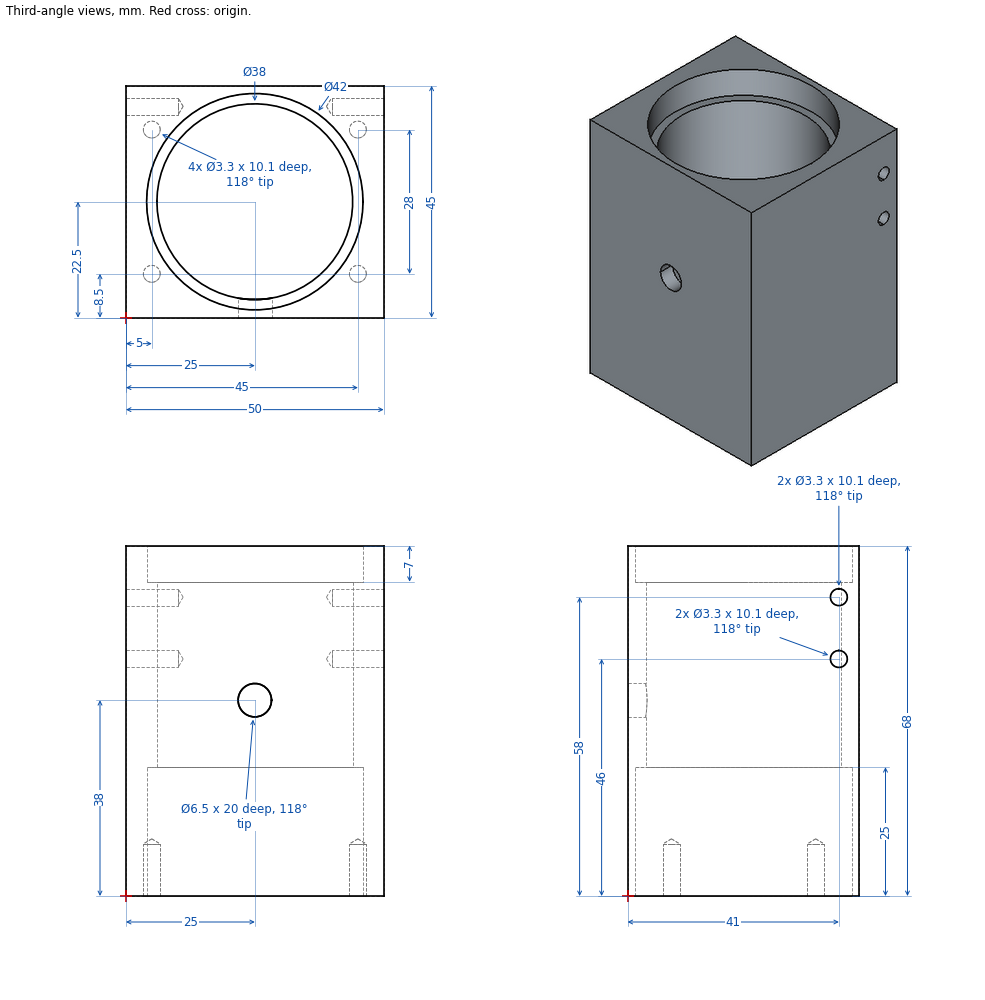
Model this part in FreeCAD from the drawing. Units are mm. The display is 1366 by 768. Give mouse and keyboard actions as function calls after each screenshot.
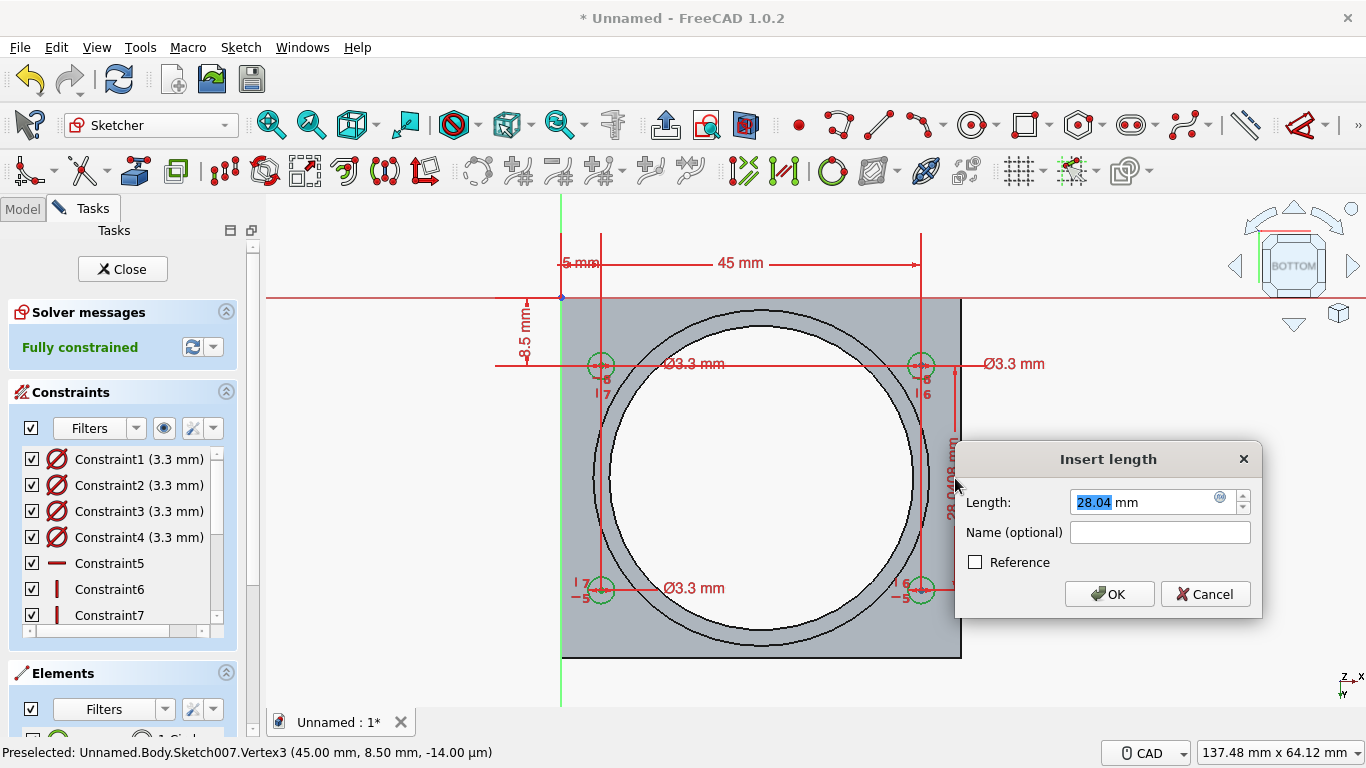
text(28)
key(Return)
key(Escape)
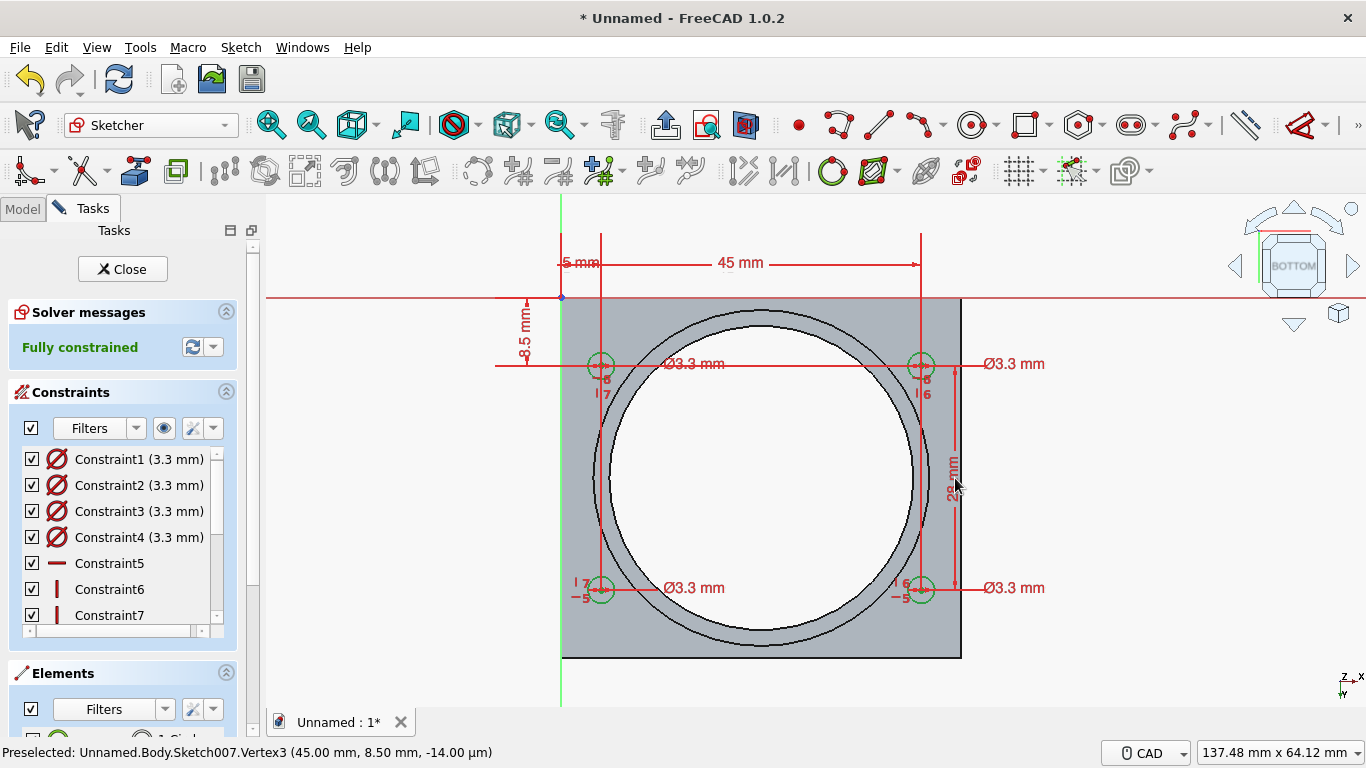
click(123, 269)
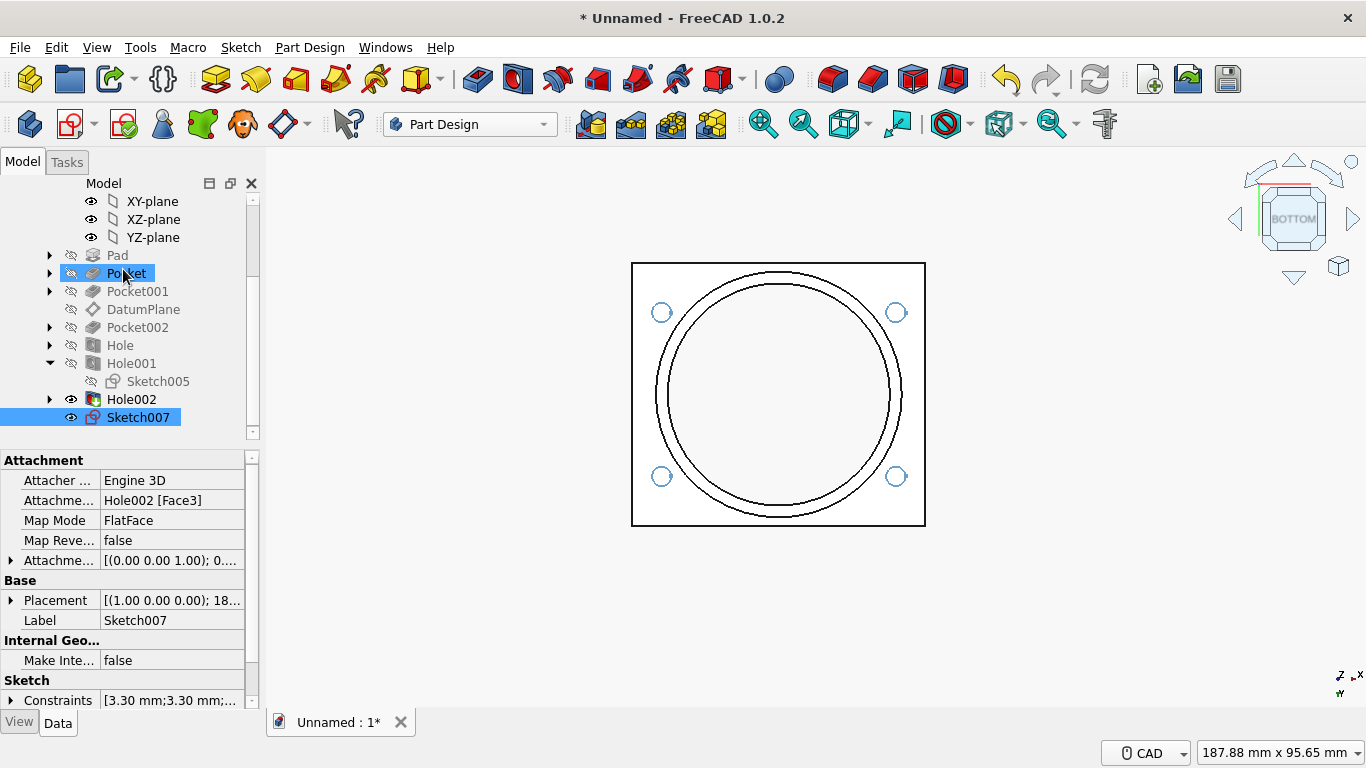
click(518, 80)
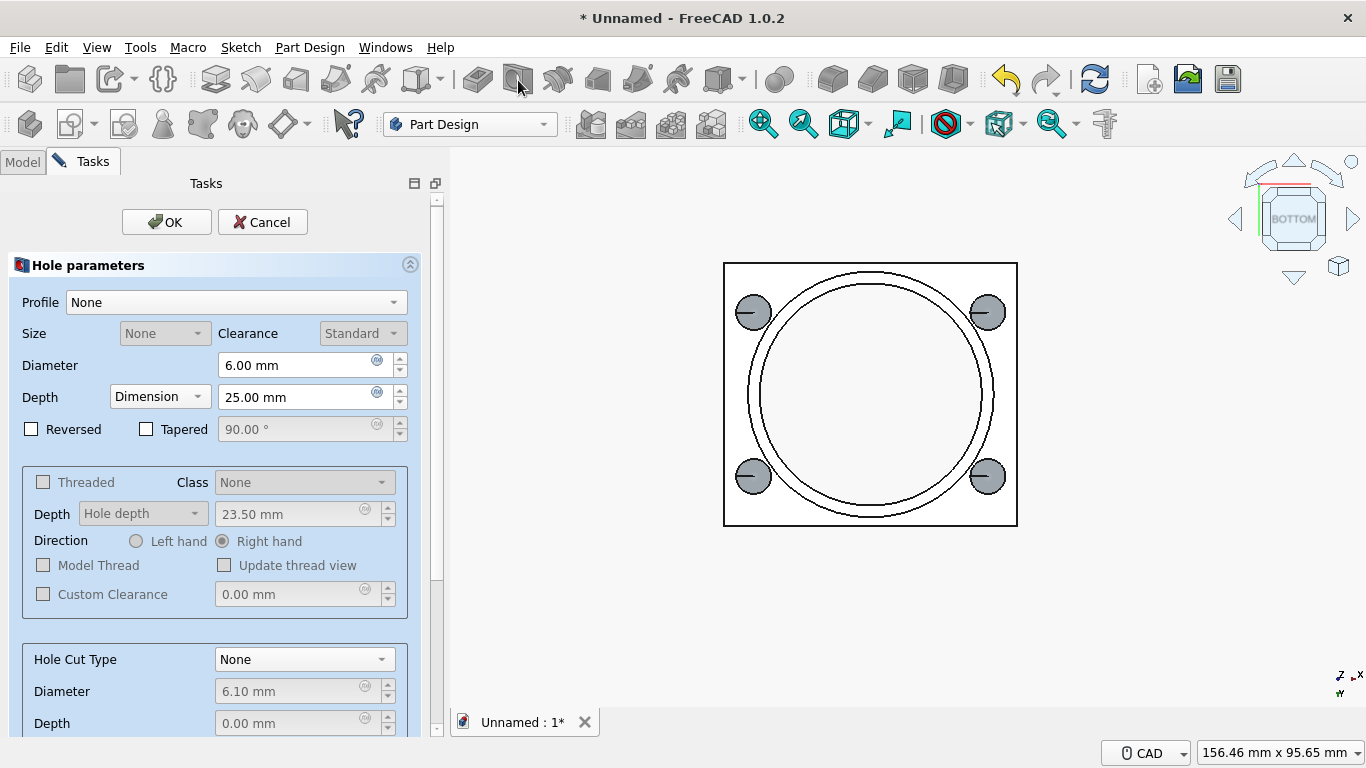
triple_click(305, 365)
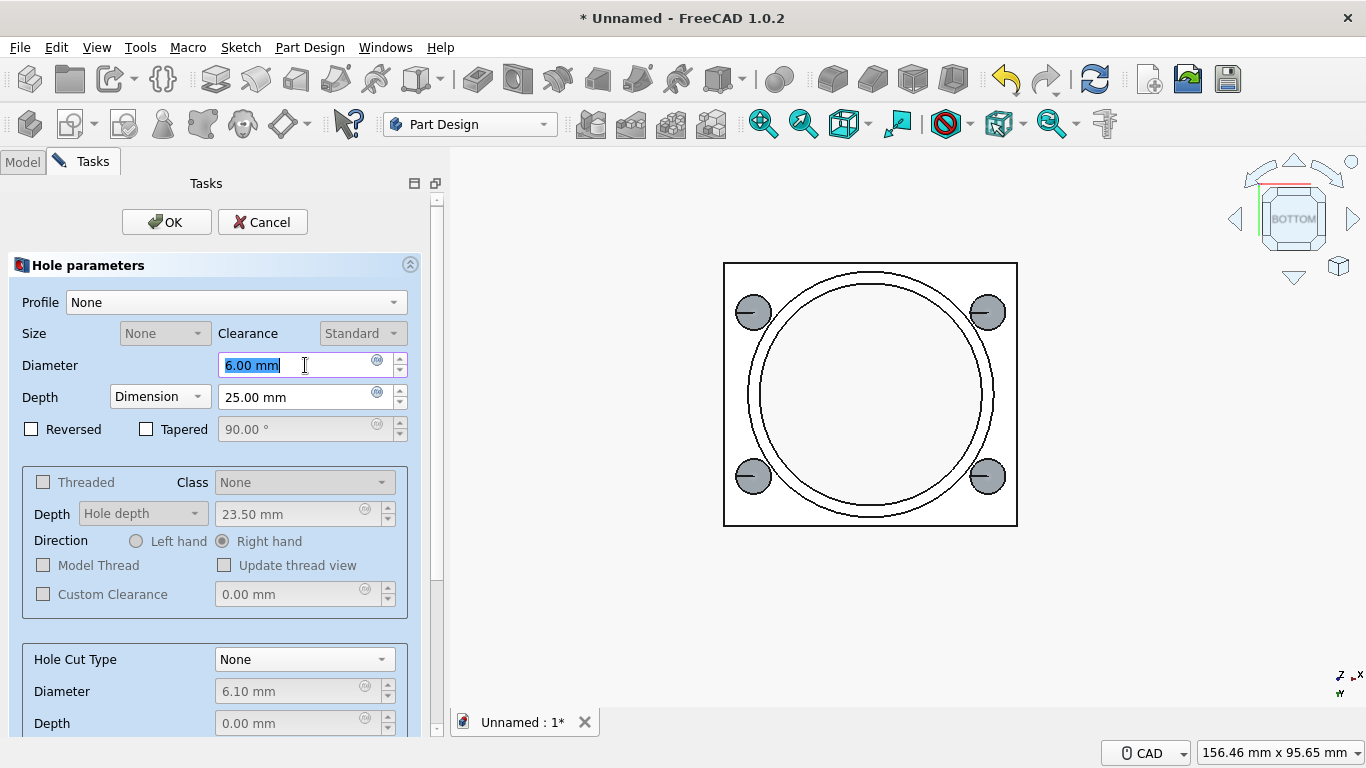
text(3.3)
key(Tab)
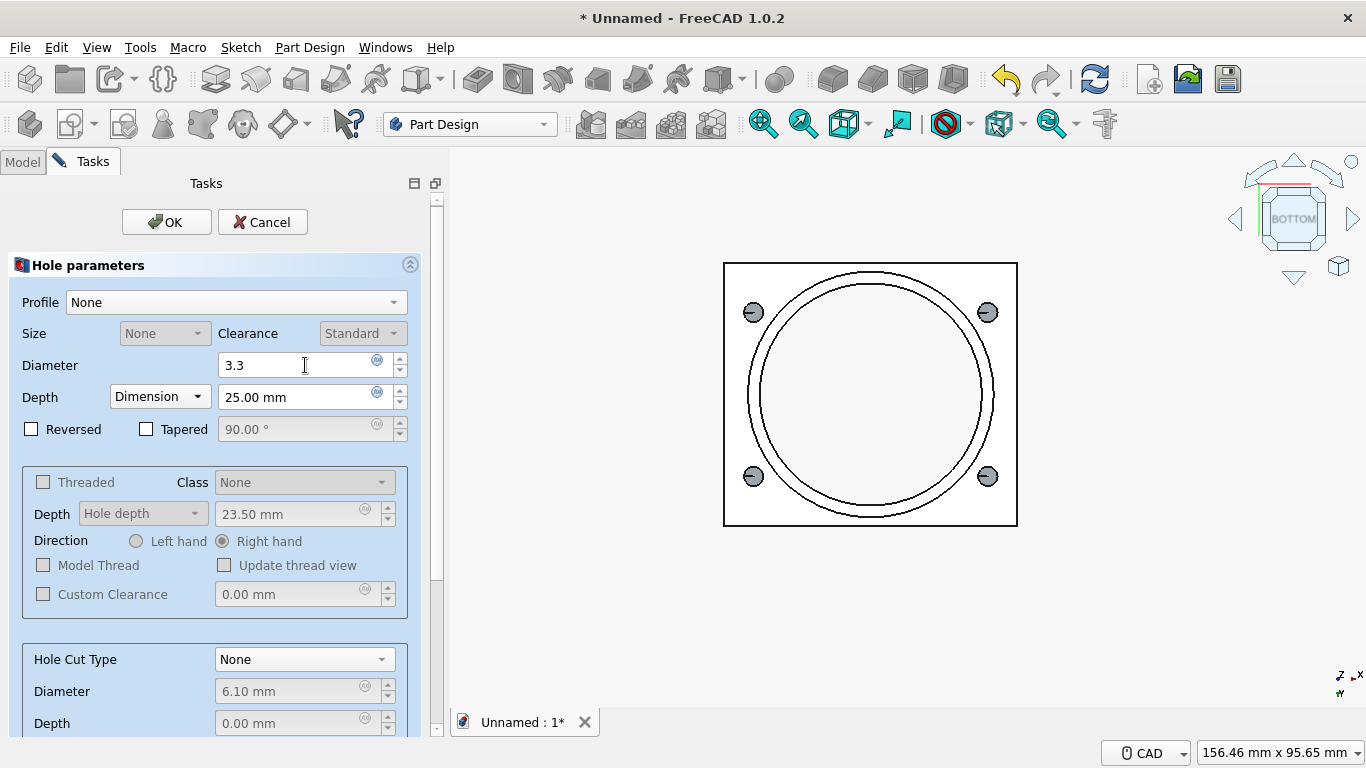
triple_click(305, 397)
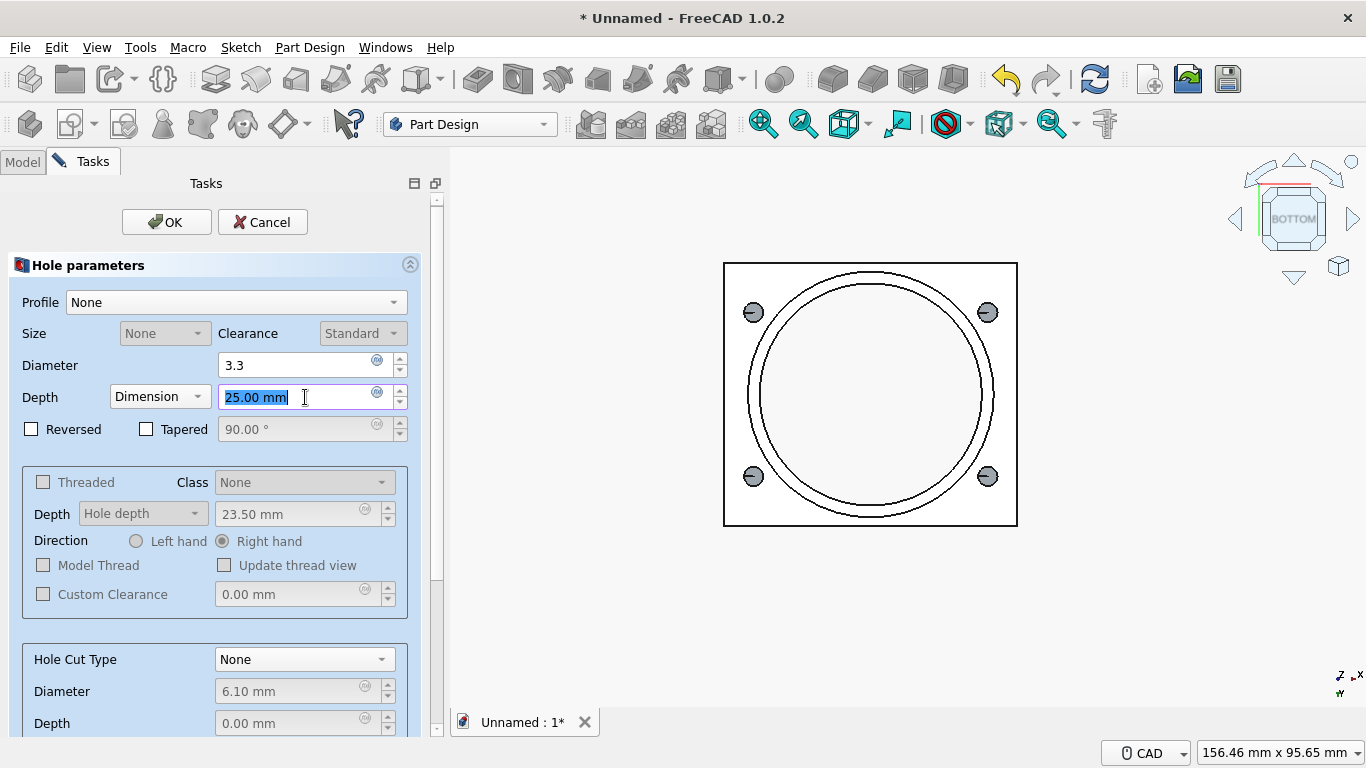
text(10.1)
key(Tab)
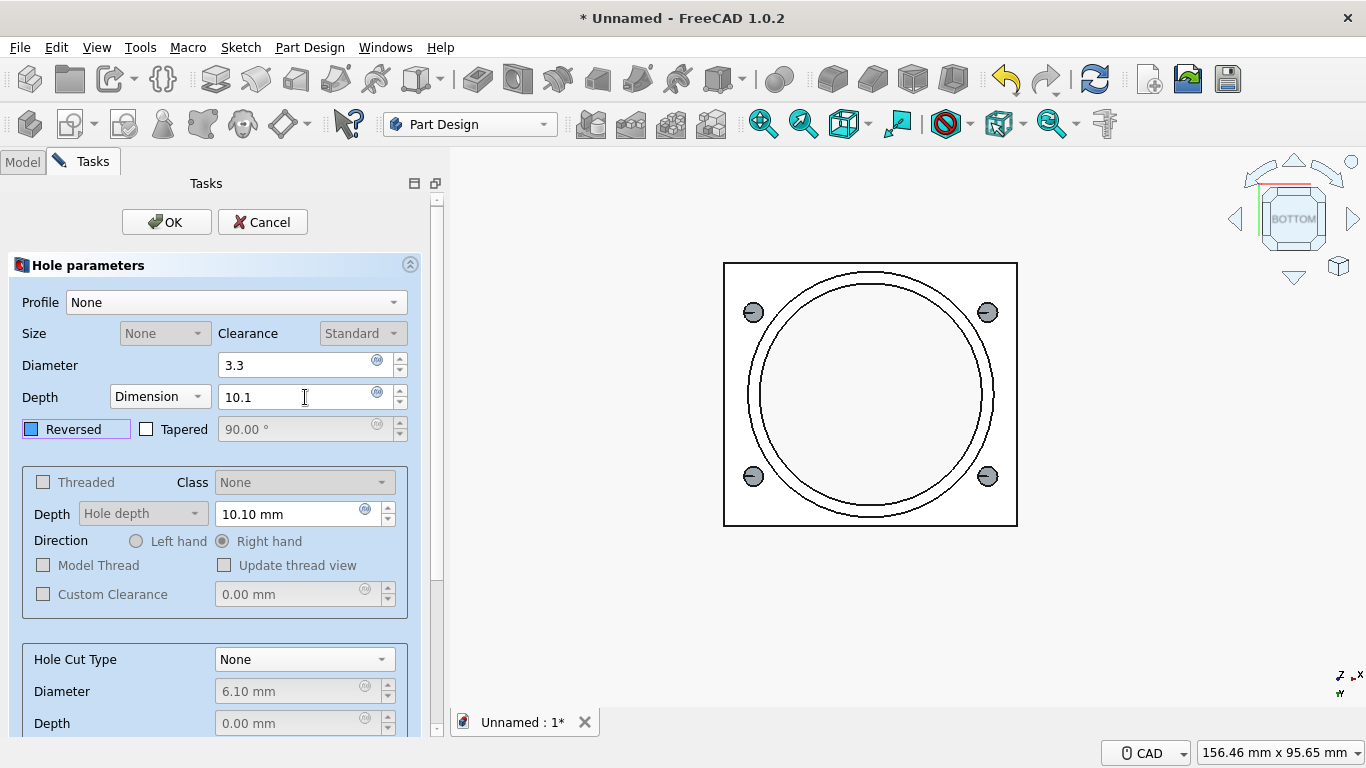
click(167, 222)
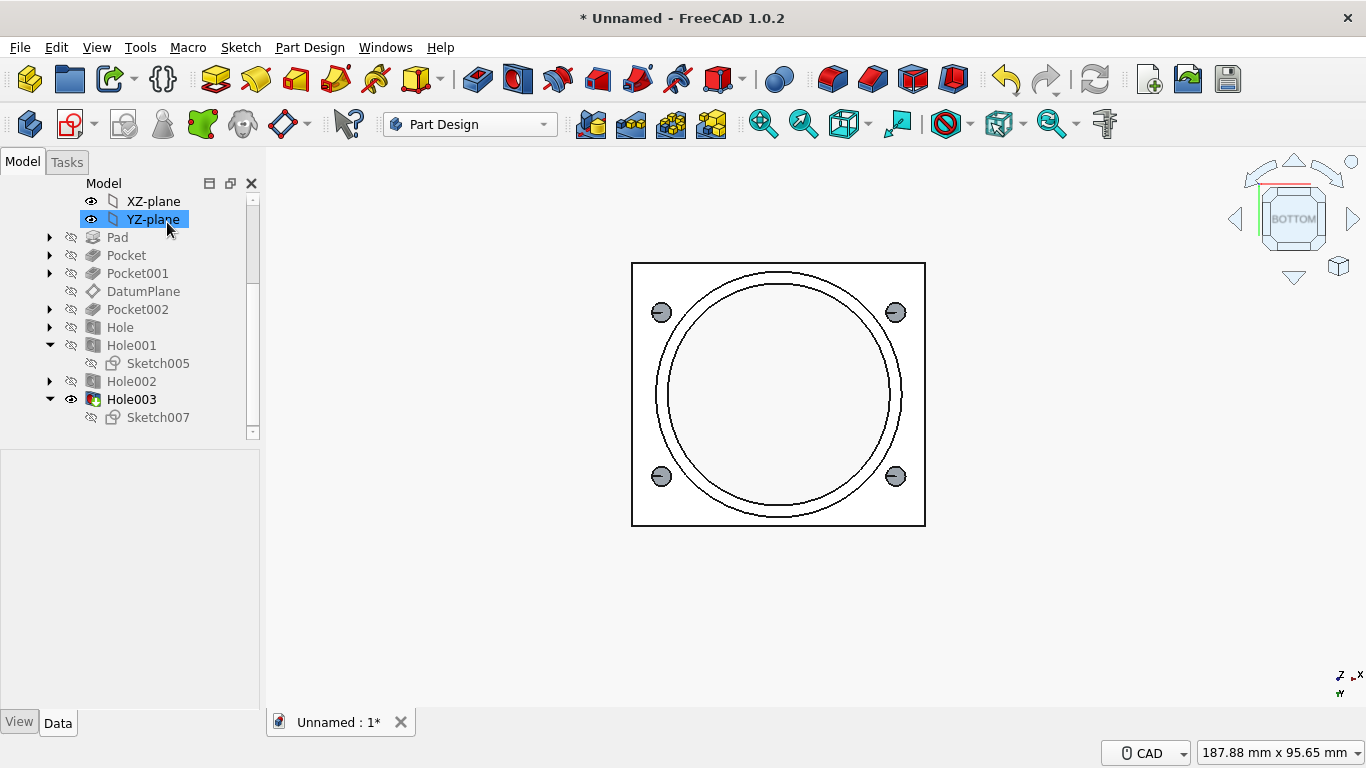
key(0)